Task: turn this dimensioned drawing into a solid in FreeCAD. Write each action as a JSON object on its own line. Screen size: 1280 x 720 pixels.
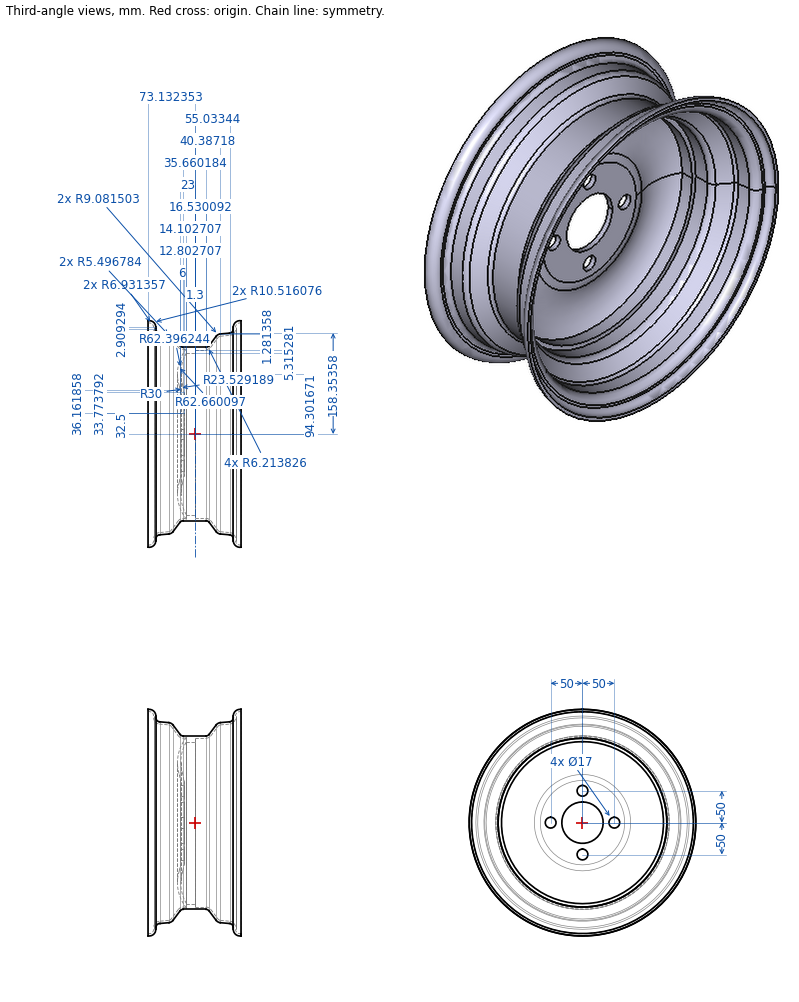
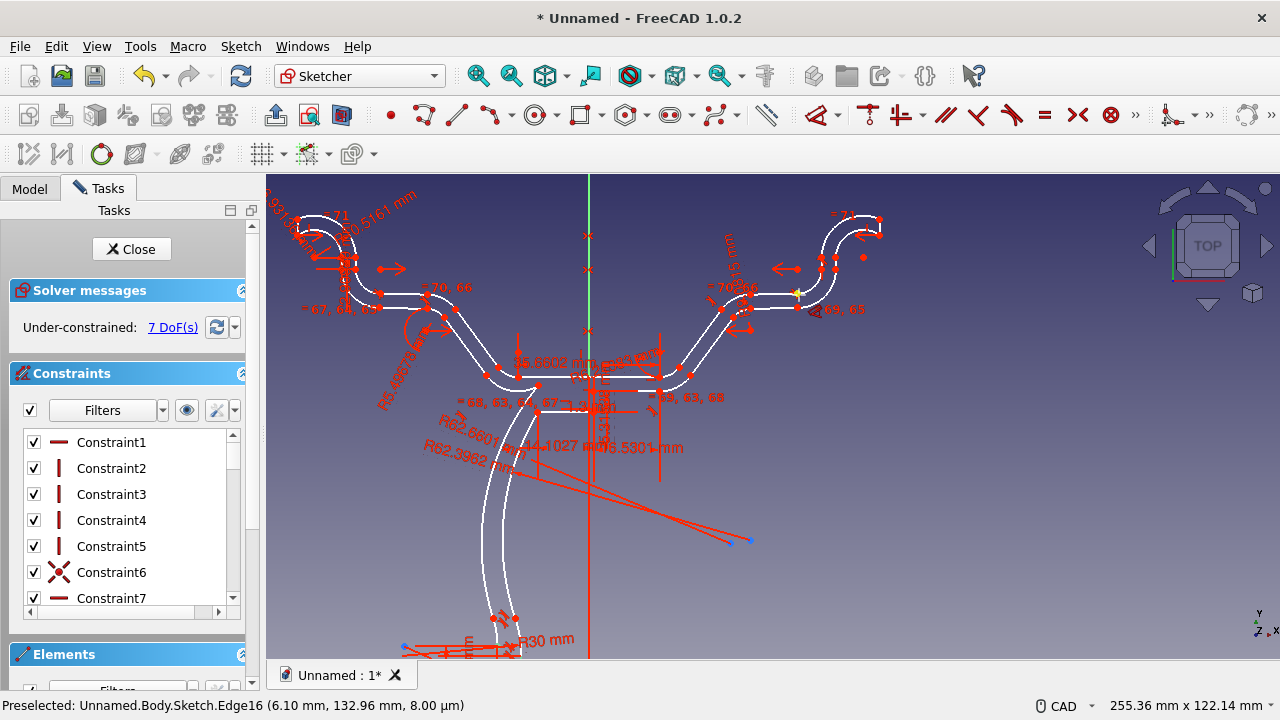
{"action": "left_click", "coordinate": [798, 294]}
{"action": "left_click", "coordinate": [645, 260]}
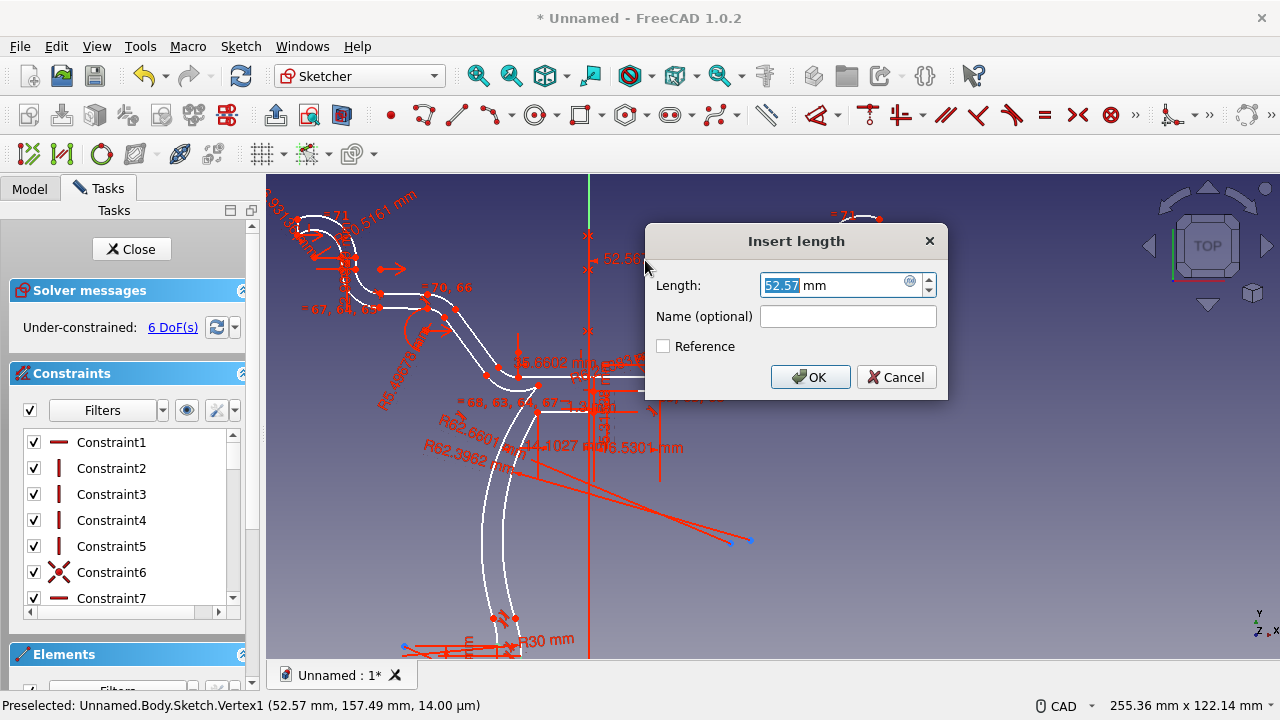
{"action": "type", "text": "55.03344"}
{"action": "key", "text": "Return"}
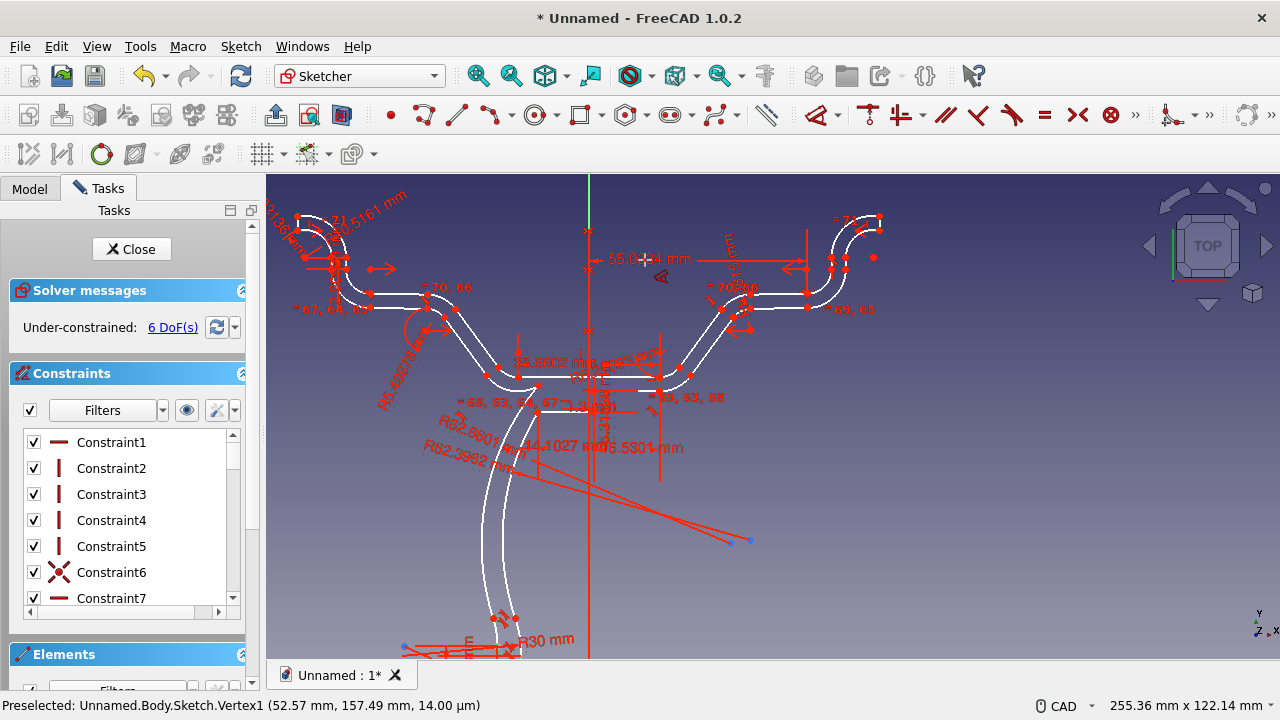
{"action": "left_click", "coordinate": [750, 295]}
{"action": "left_click", "coordinate": [670, 237]}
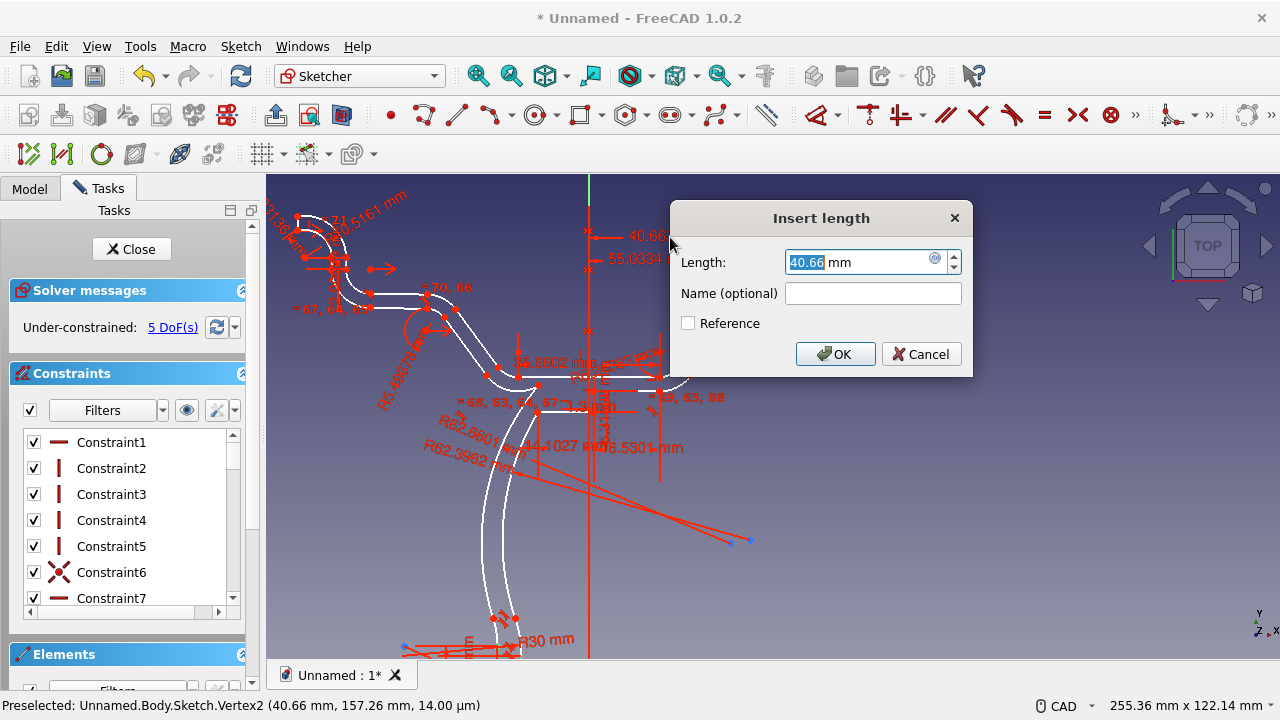
{"action": "type", "text": "40.38718"}
{"action": "key", "text": "Return"}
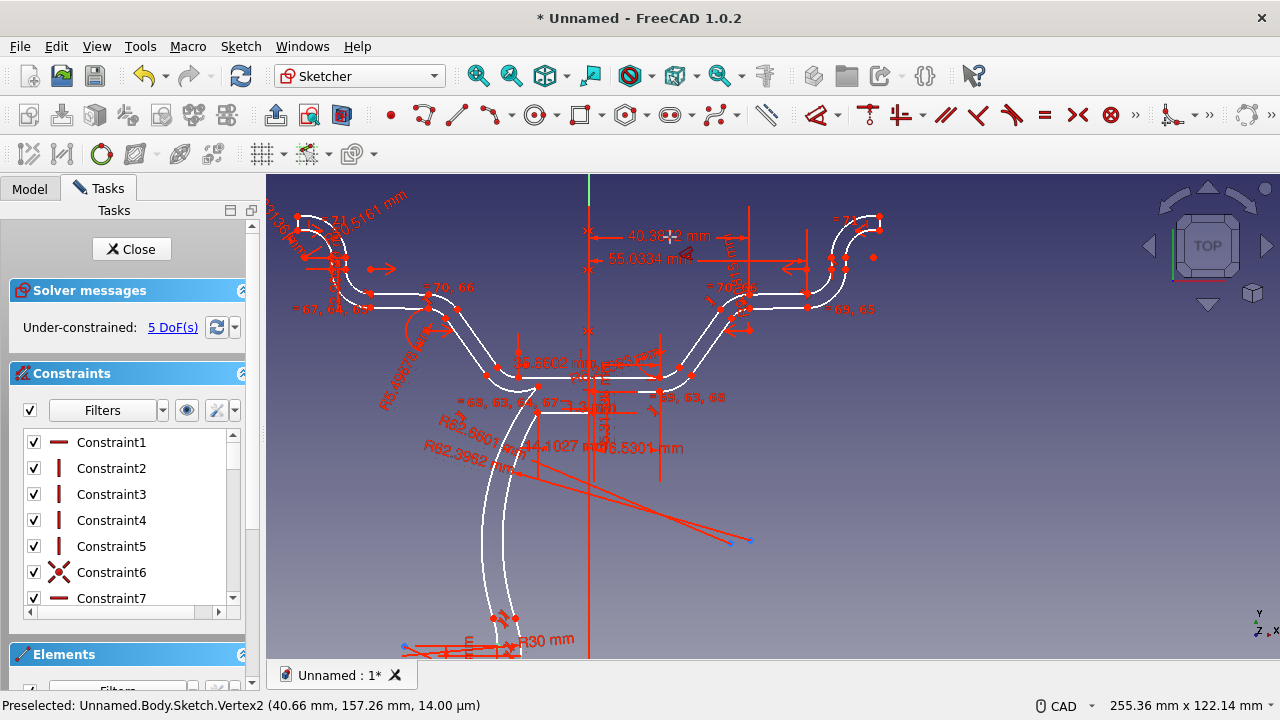
{"action": "scroll", "coordinate": [790, 294], "scroll_direction": "up", "scroll_amount": 11}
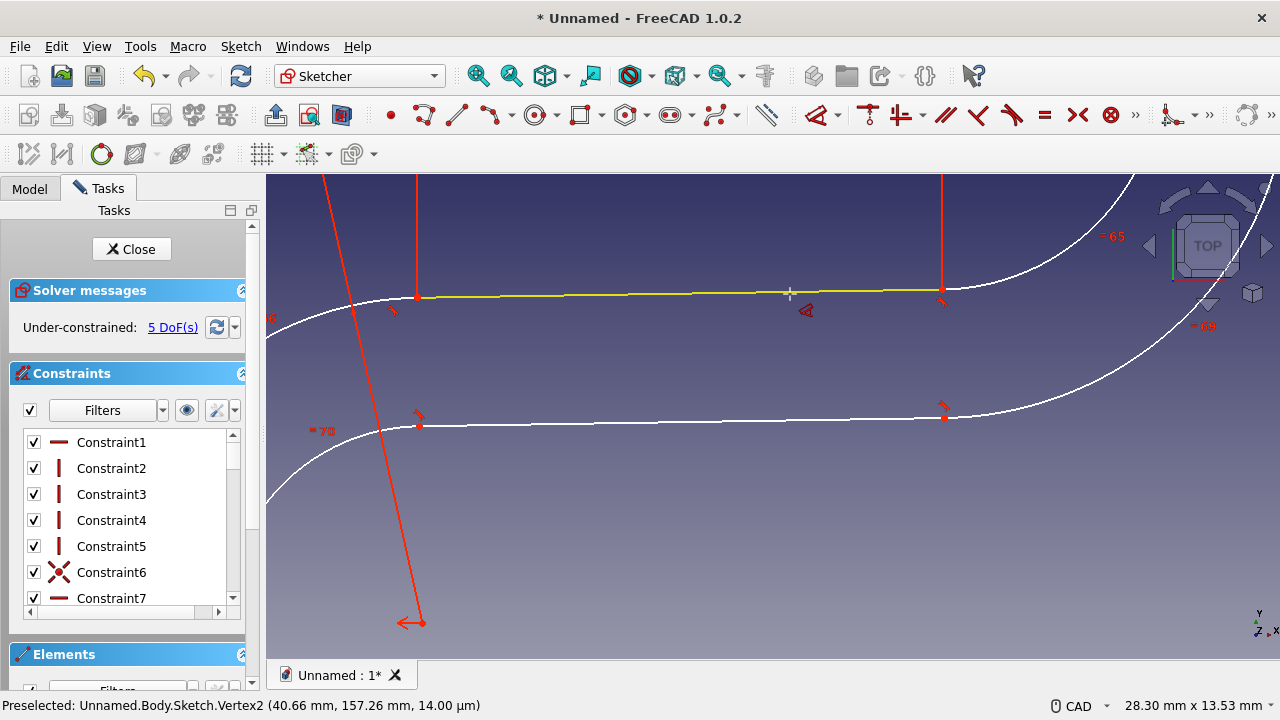
{"action": "left_click", "coordinate": [785, 292]}
{"action": "left_click", "coordinate": [1000, 296]}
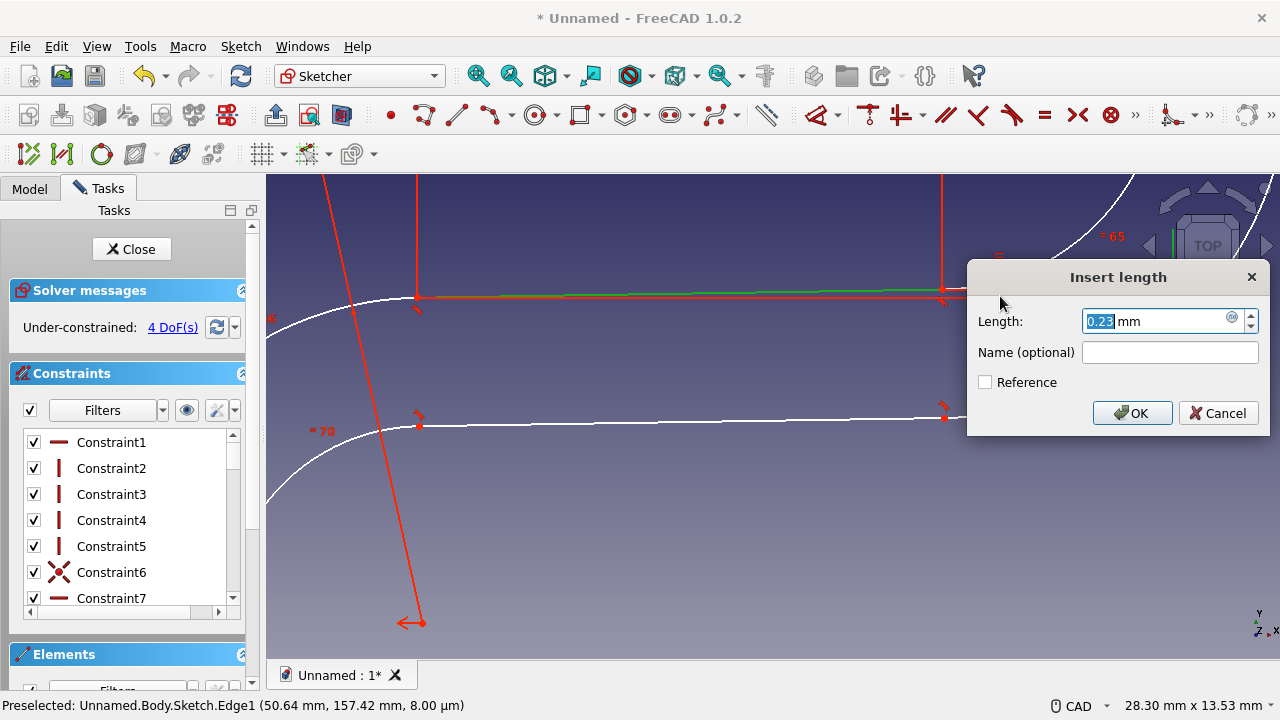
{"action": "type", "text": "1.281358"}
{"action": "key", "text": "Return"}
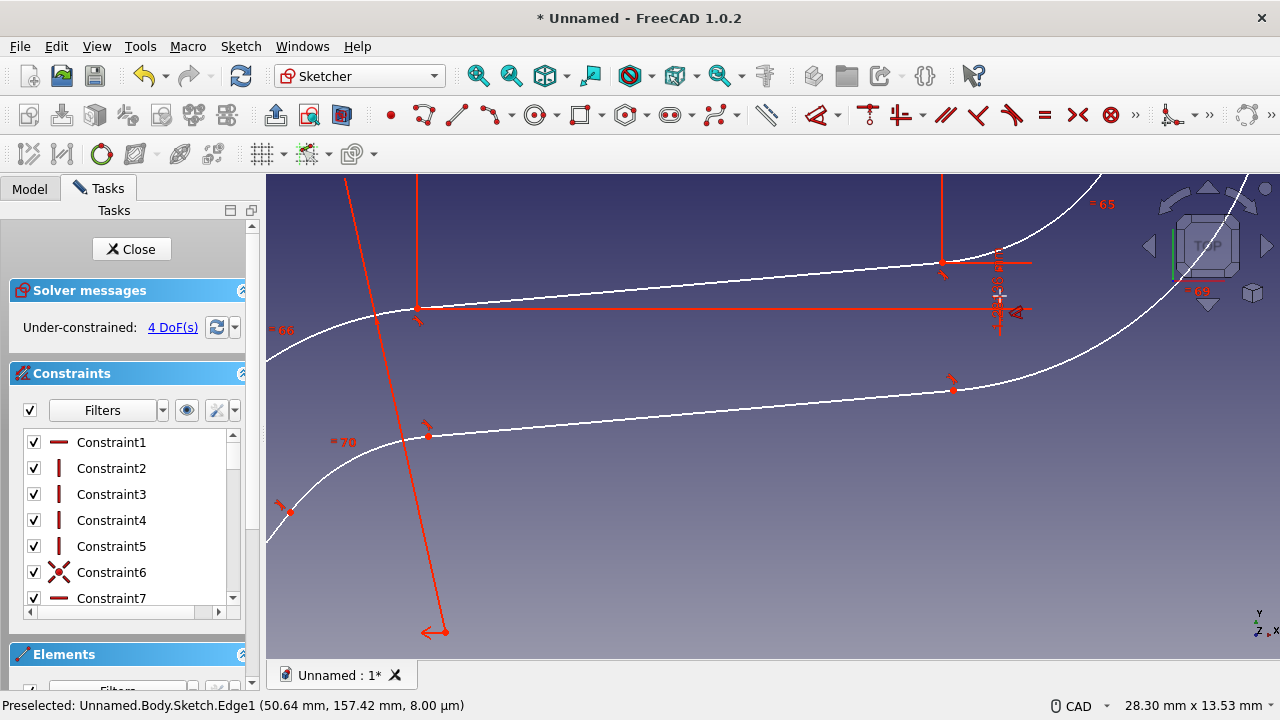
{"action": "scroll", "coordinate": [795, 294], "scroll_direction": "down", "scroll_amount": 15}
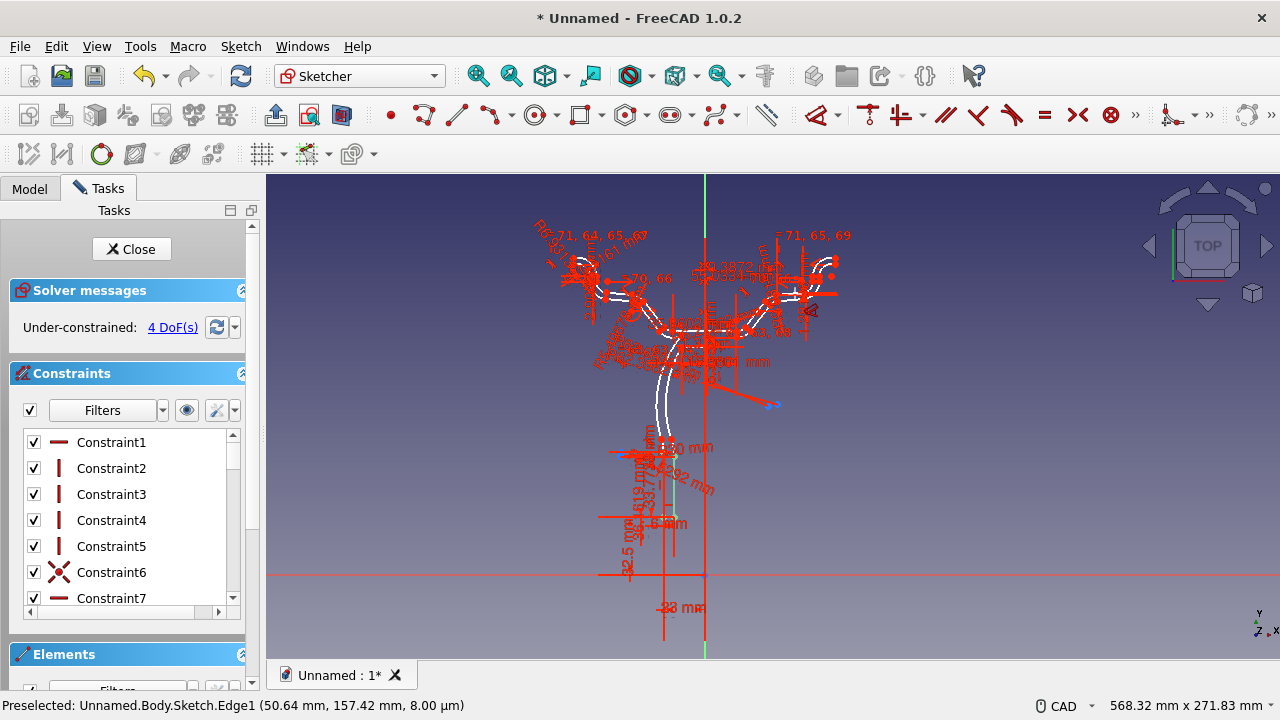
{"action": "scroll", "coordinate": [803, 293], "scroll_direction": "up", "scroll_amount": 4}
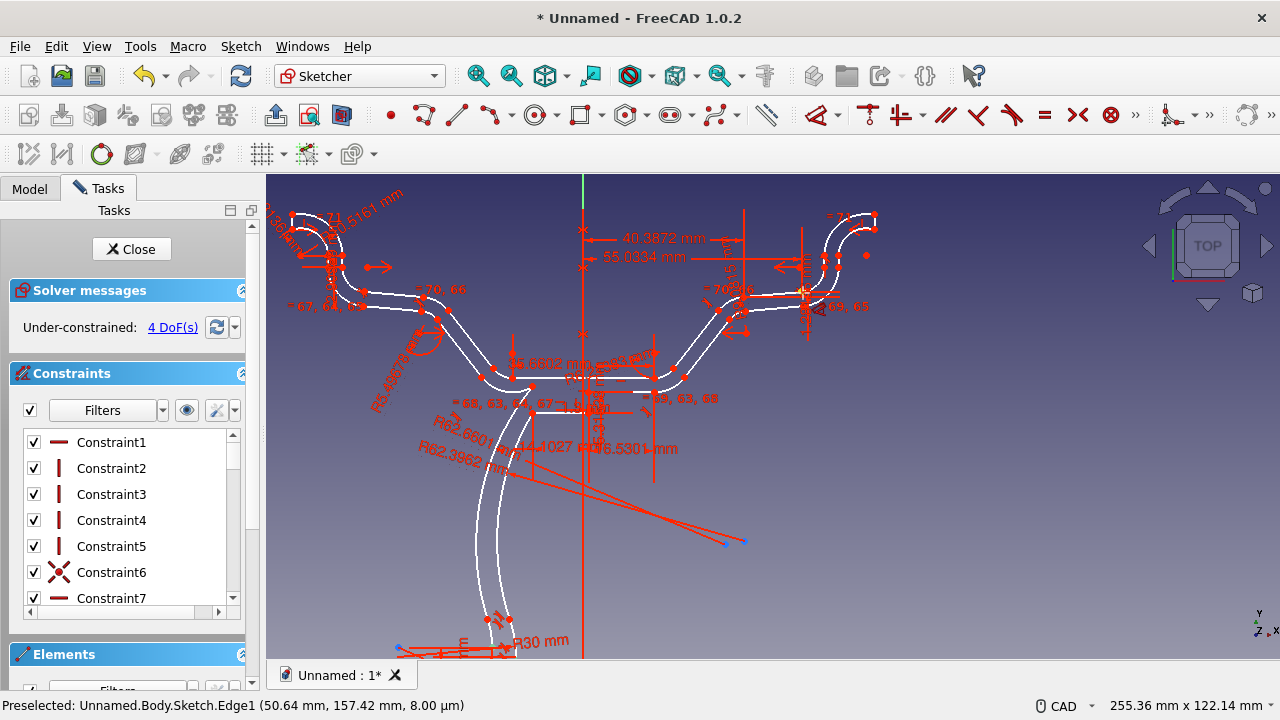
{"action": "left_click", "coordinate": [802, 292]}
{"action": "left_click", "coordinate": [836, 461]}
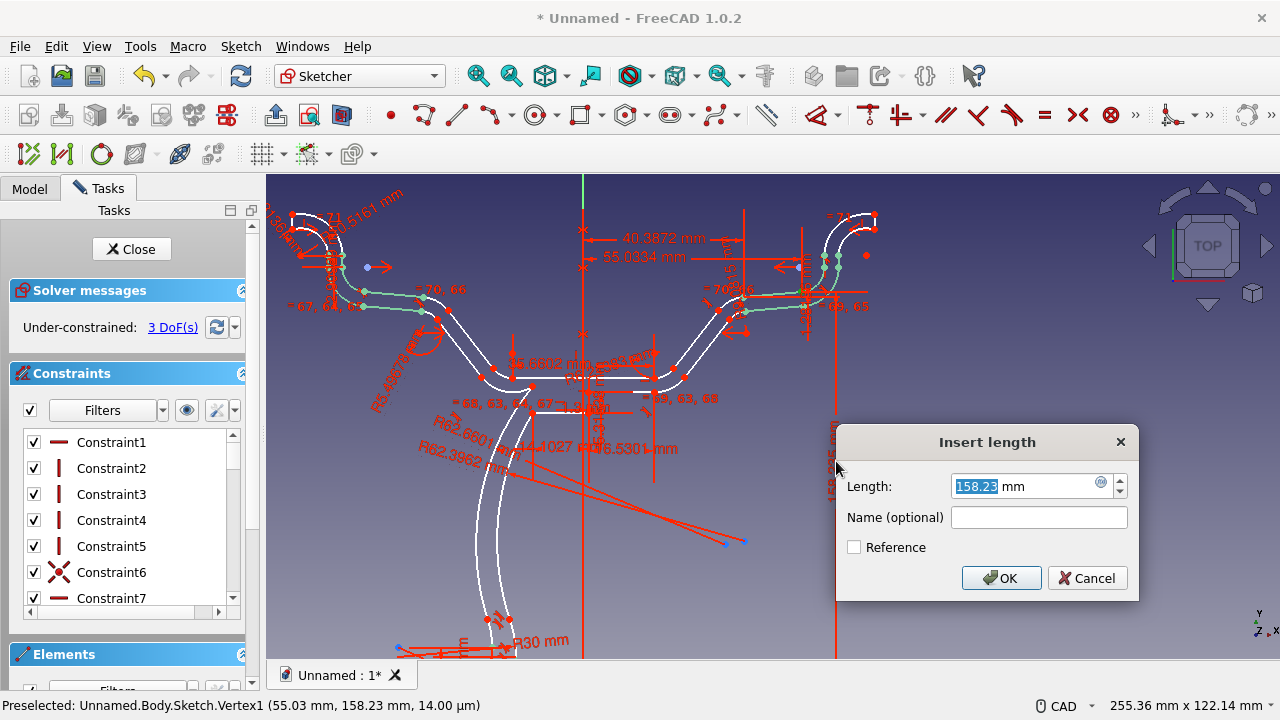
{"action": "type", "text": "158.35358"}
{"action": "key", "text": "Return"}